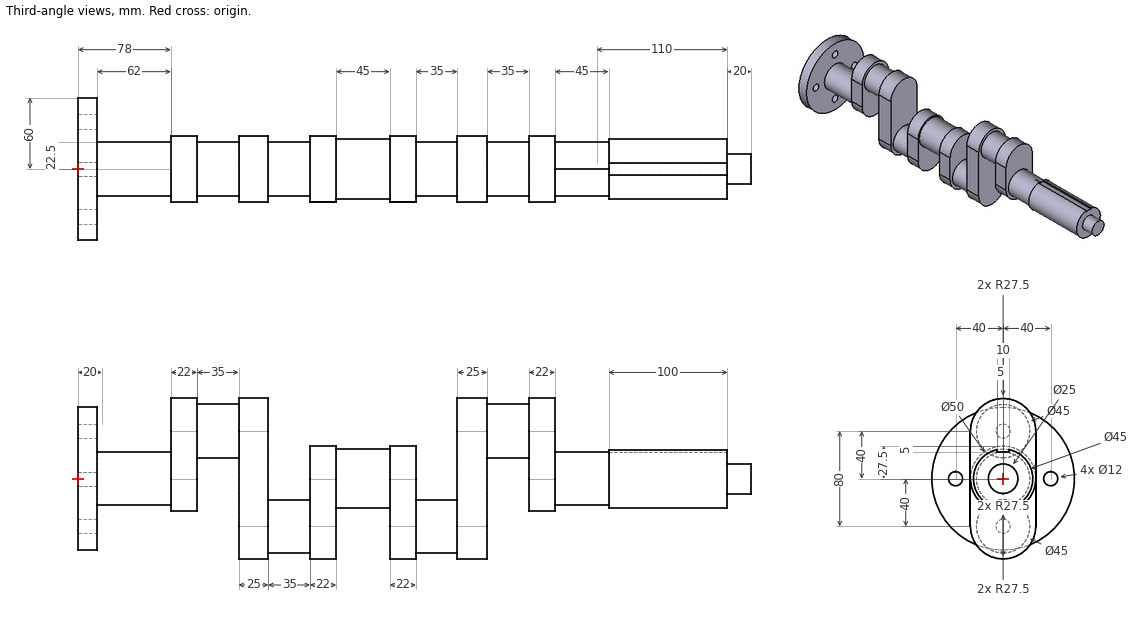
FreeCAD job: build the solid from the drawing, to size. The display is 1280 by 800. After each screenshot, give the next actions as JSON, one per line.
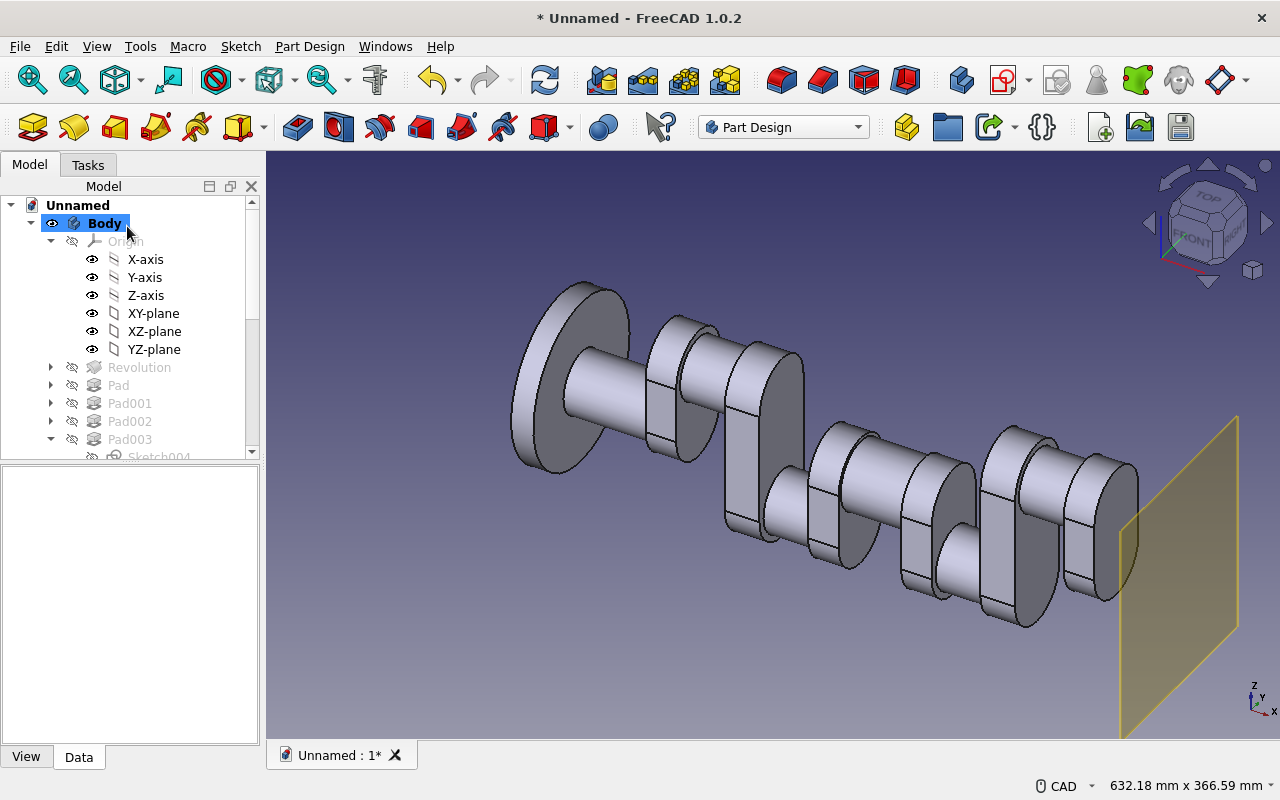
{"action": "scroll", "coordinate": [101, 327], "scroll_direction": "down", "scroll_amount": 3}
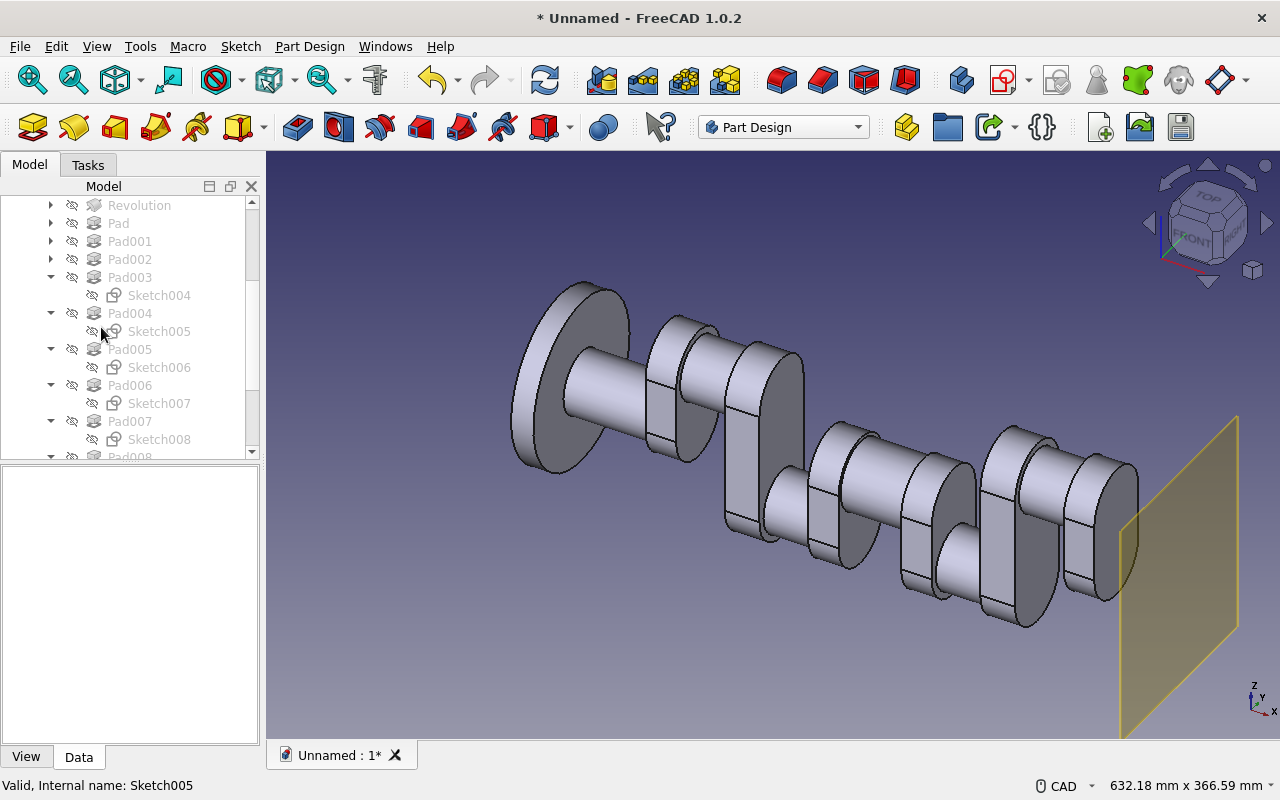
{"action": "scroll", "coordinate": [141, 327], "scroll_direction": "up", "scroll_amount": 15}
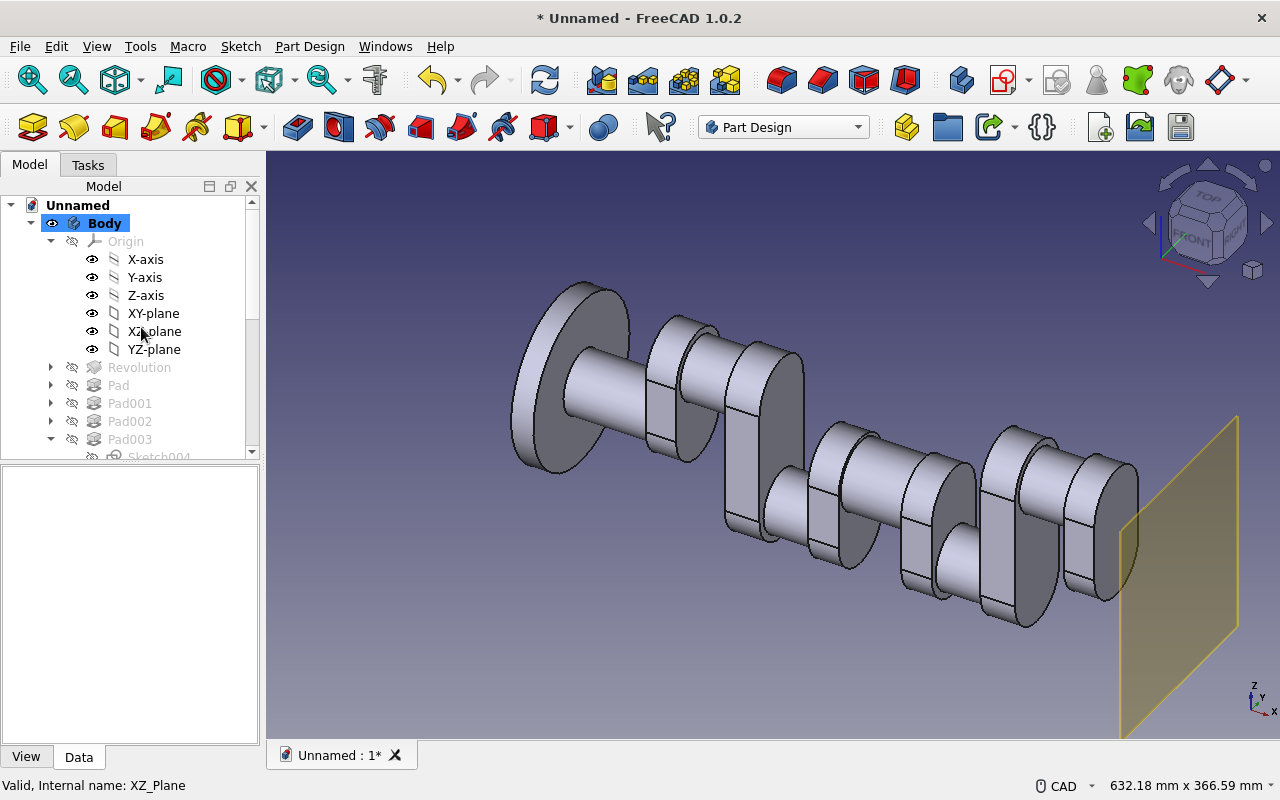
{"action": "scroll", "coordinate": [101, 327], "scroll_direction": "down", "scroll_amount": 6}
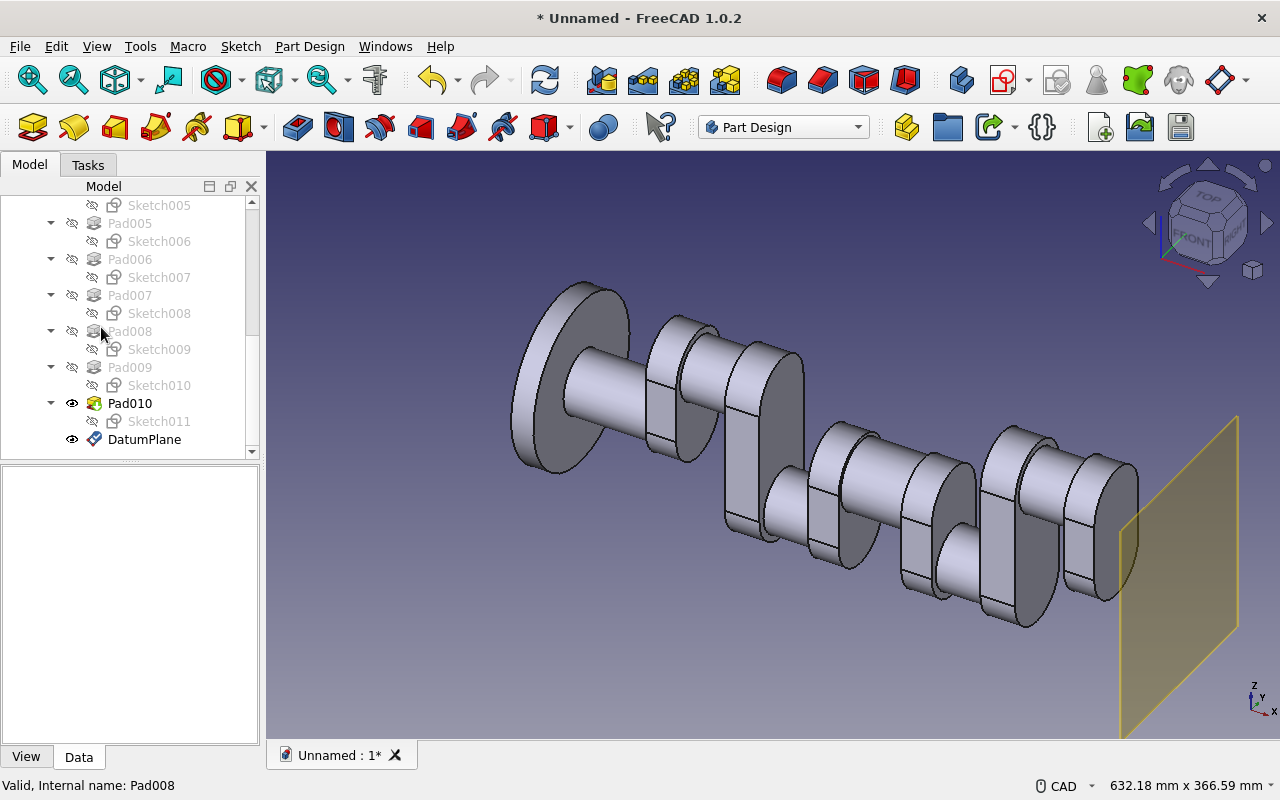
{"action": "left_click", "coordinate": [117, 439]}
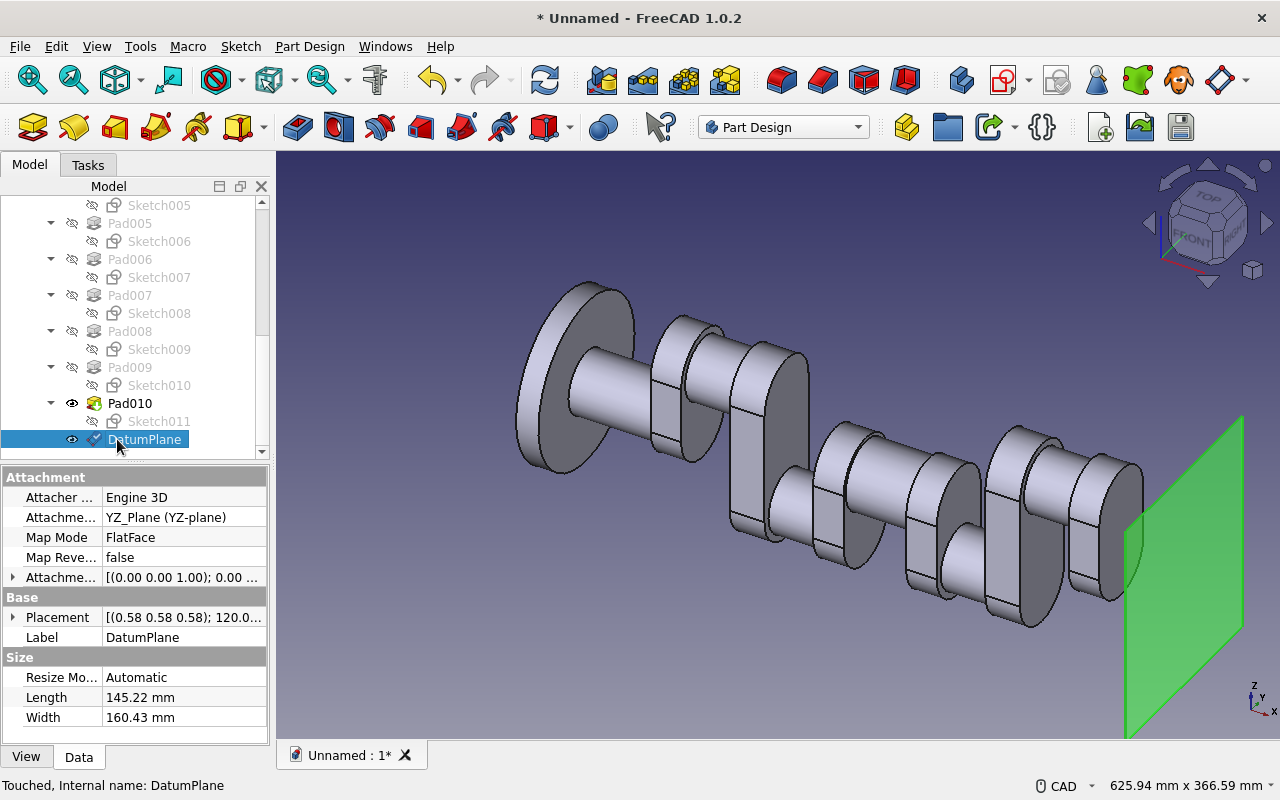
{"action": "left_click", "coordinate": [1002, 80]}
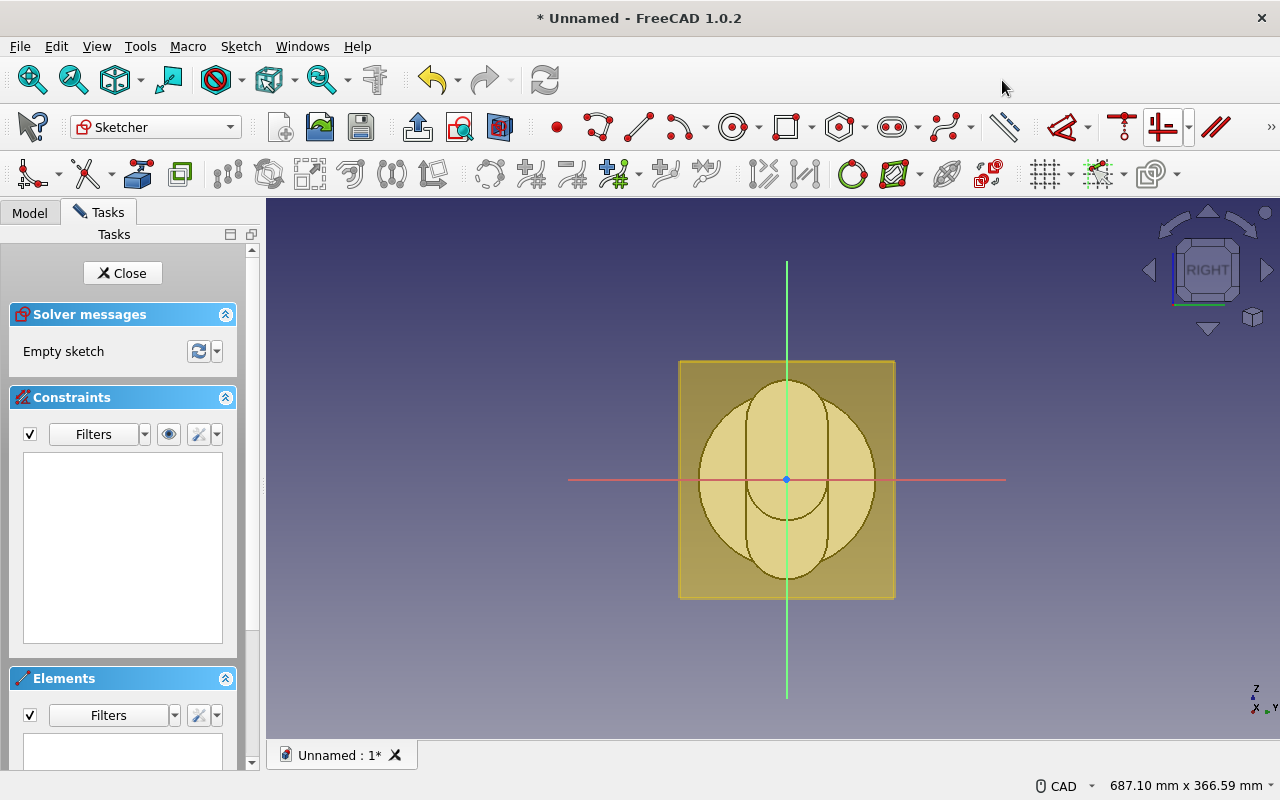
{"action": "scroll", "coordinate": [808, 483], "scroll_direction": "up", "scroll_amount": 8}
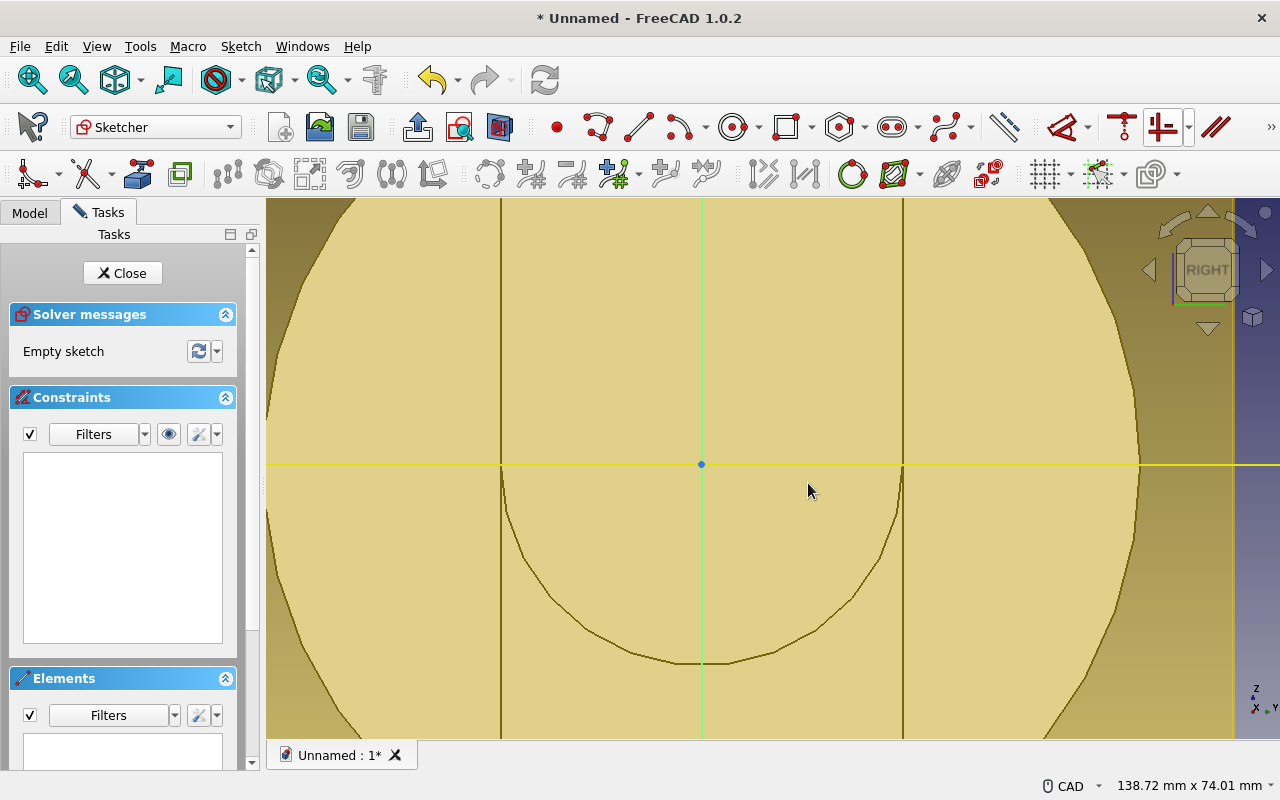
{"action": "left_click", "coordinate": [732, 128]}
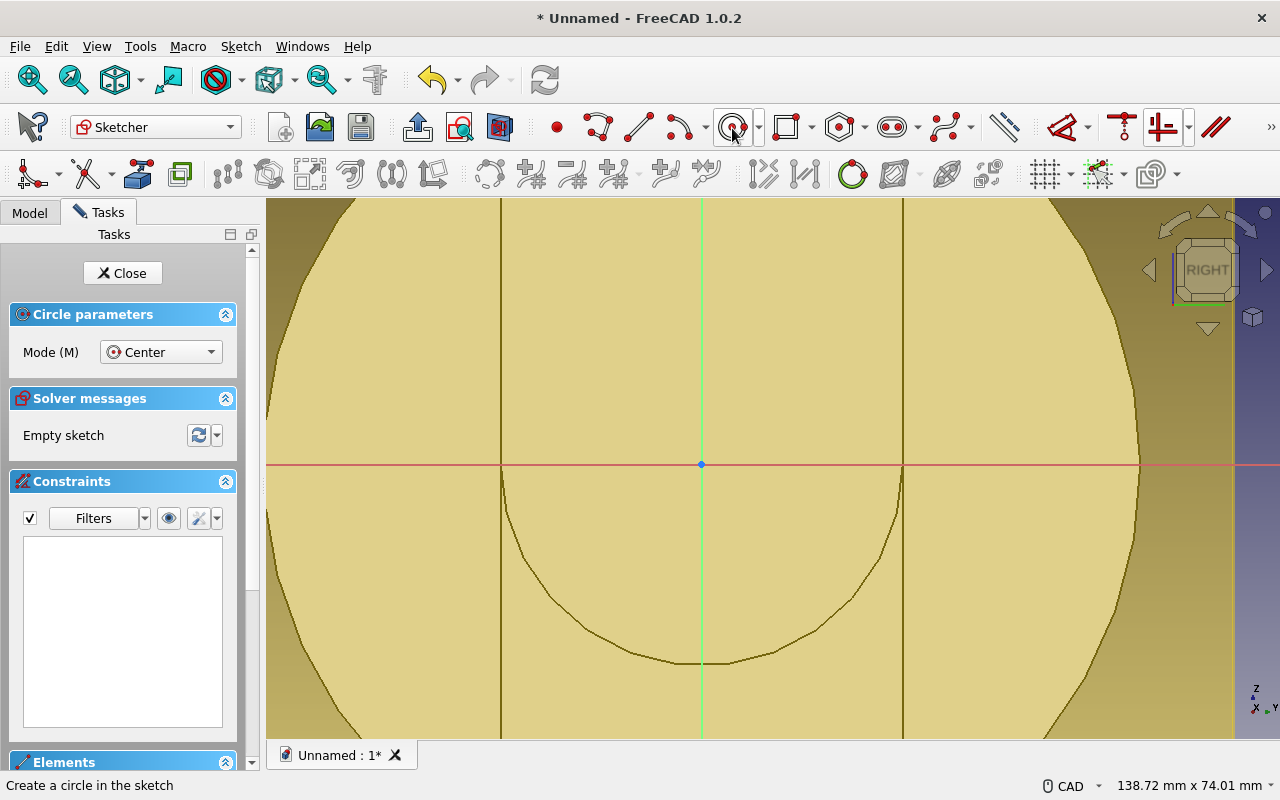
{"action": "left_click", "coordinate": [702, 465]}
{"action": "left_click", "coordinate": [818, 349]}
{"action": "key", "text": "Escape"}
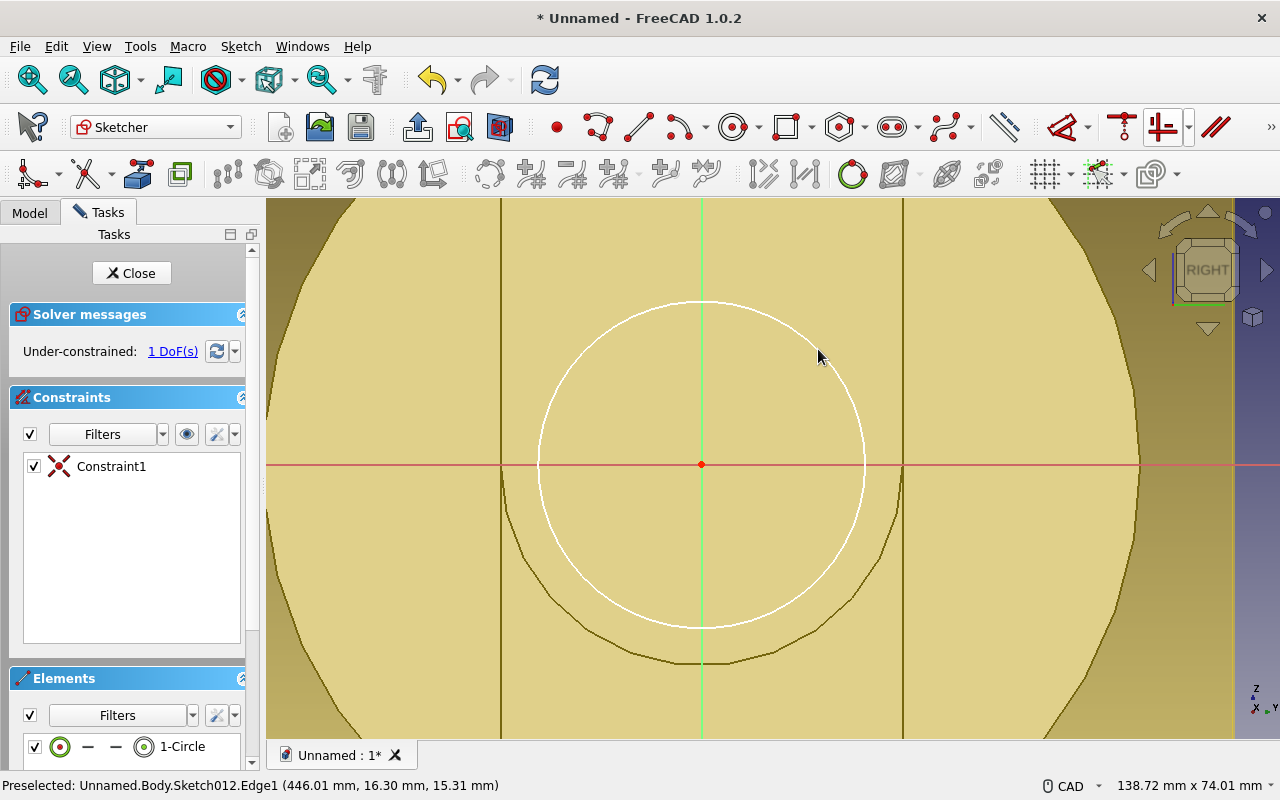
{"action": "left_click", "coordinate": [1062, 128]}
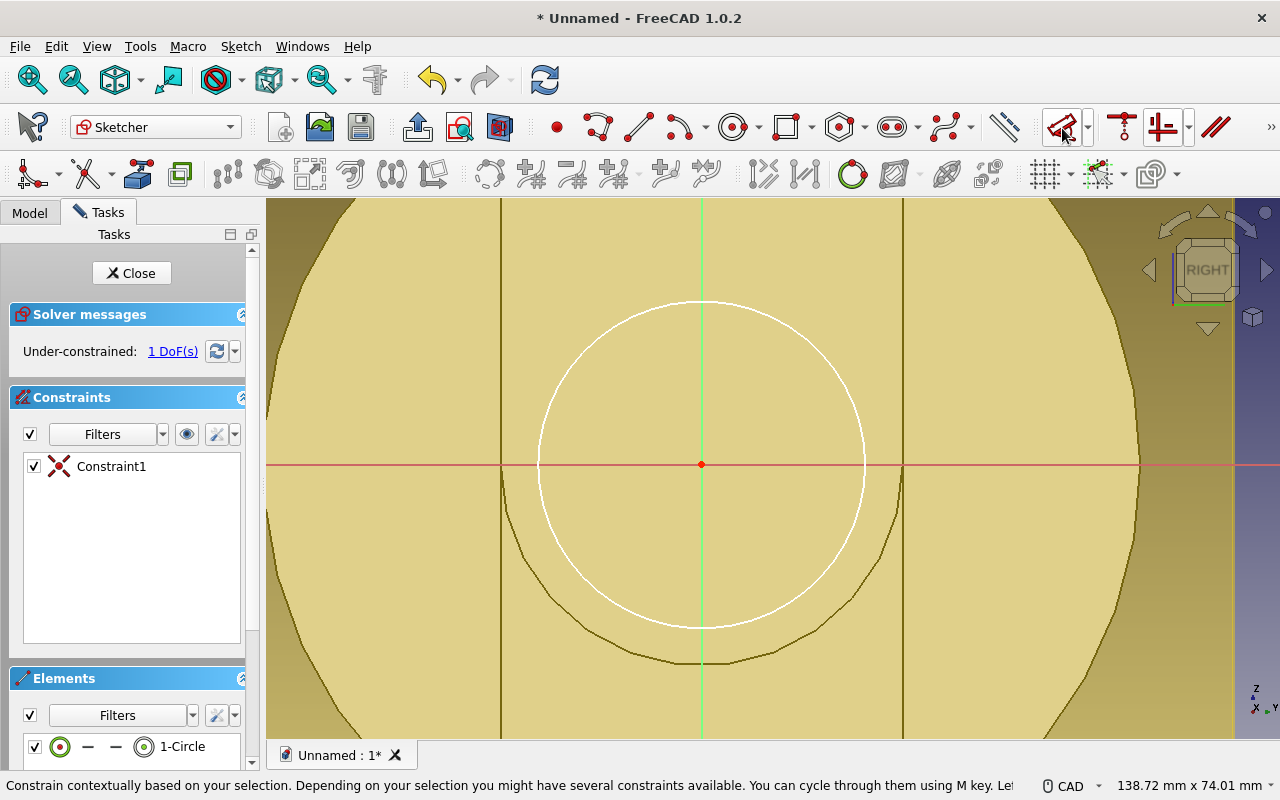
{"action": "left_click", "coordinate": [817, 349]}
{"action": "left_click", "coordinate": [840, 326]}